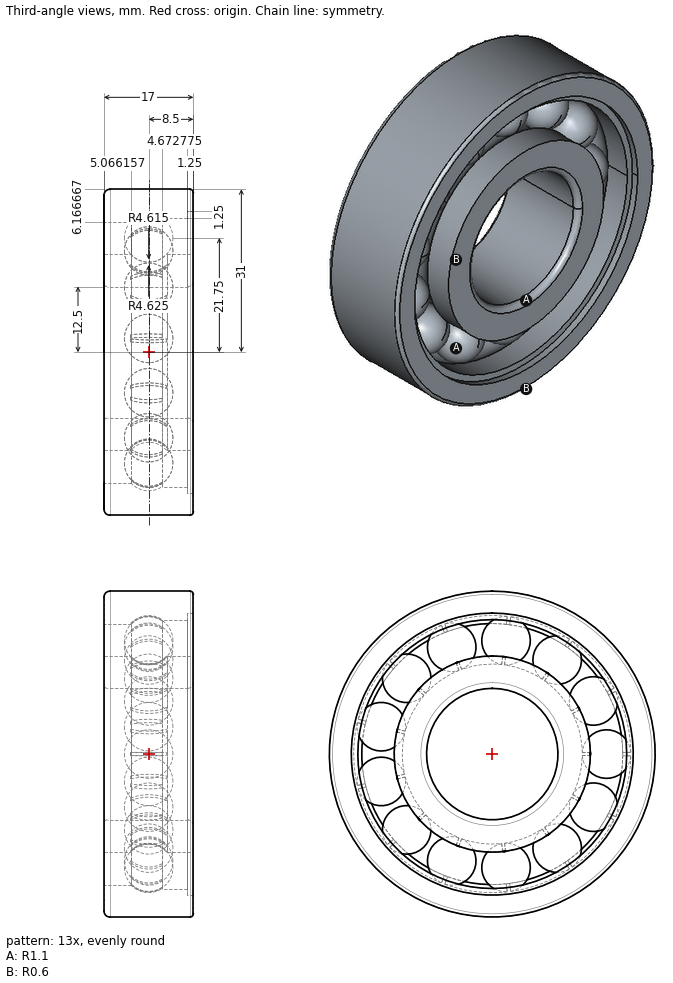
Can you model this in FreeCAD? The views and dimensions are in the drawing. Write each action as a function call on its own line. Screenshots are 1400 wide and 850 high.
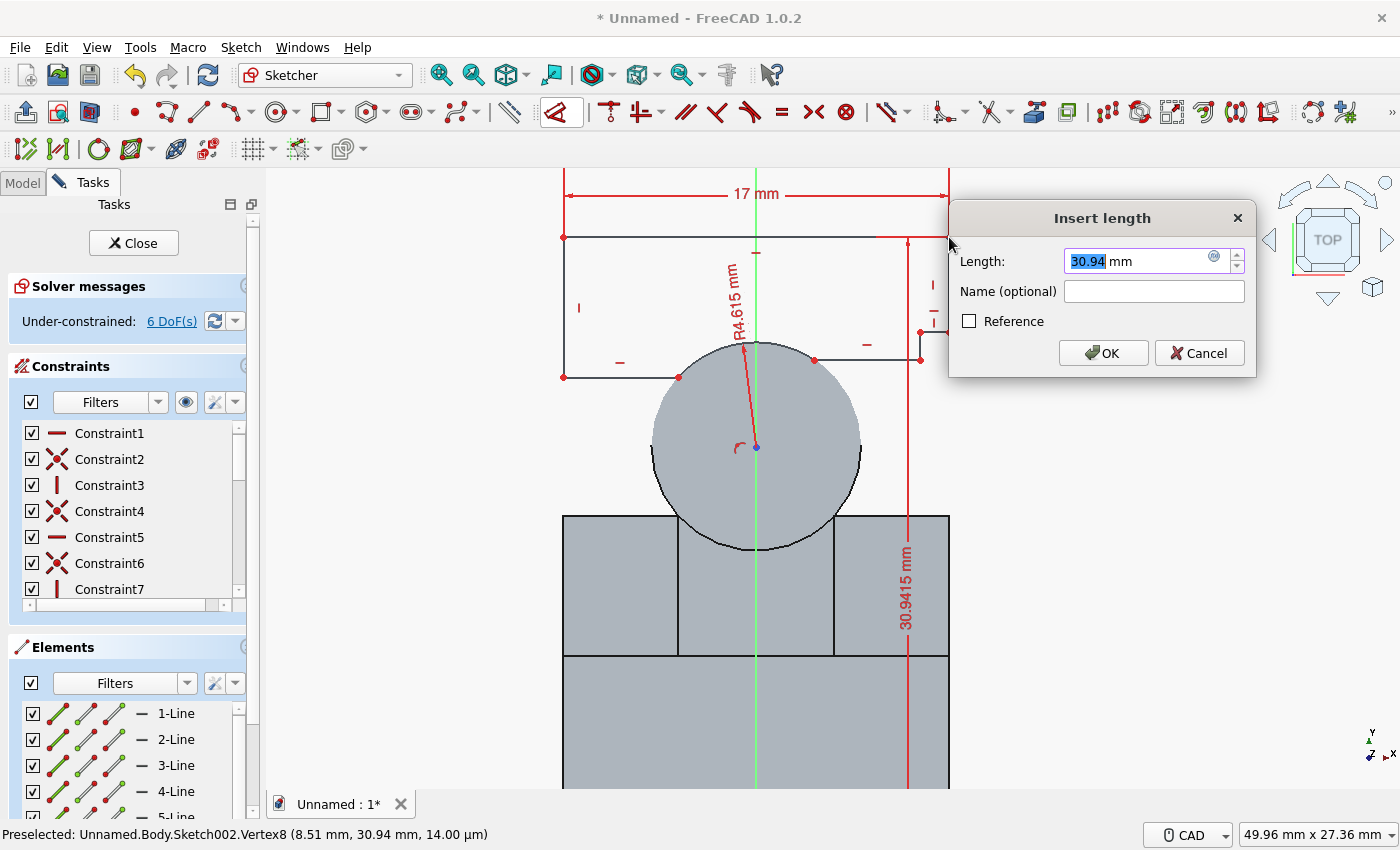
text(31)
key(Return)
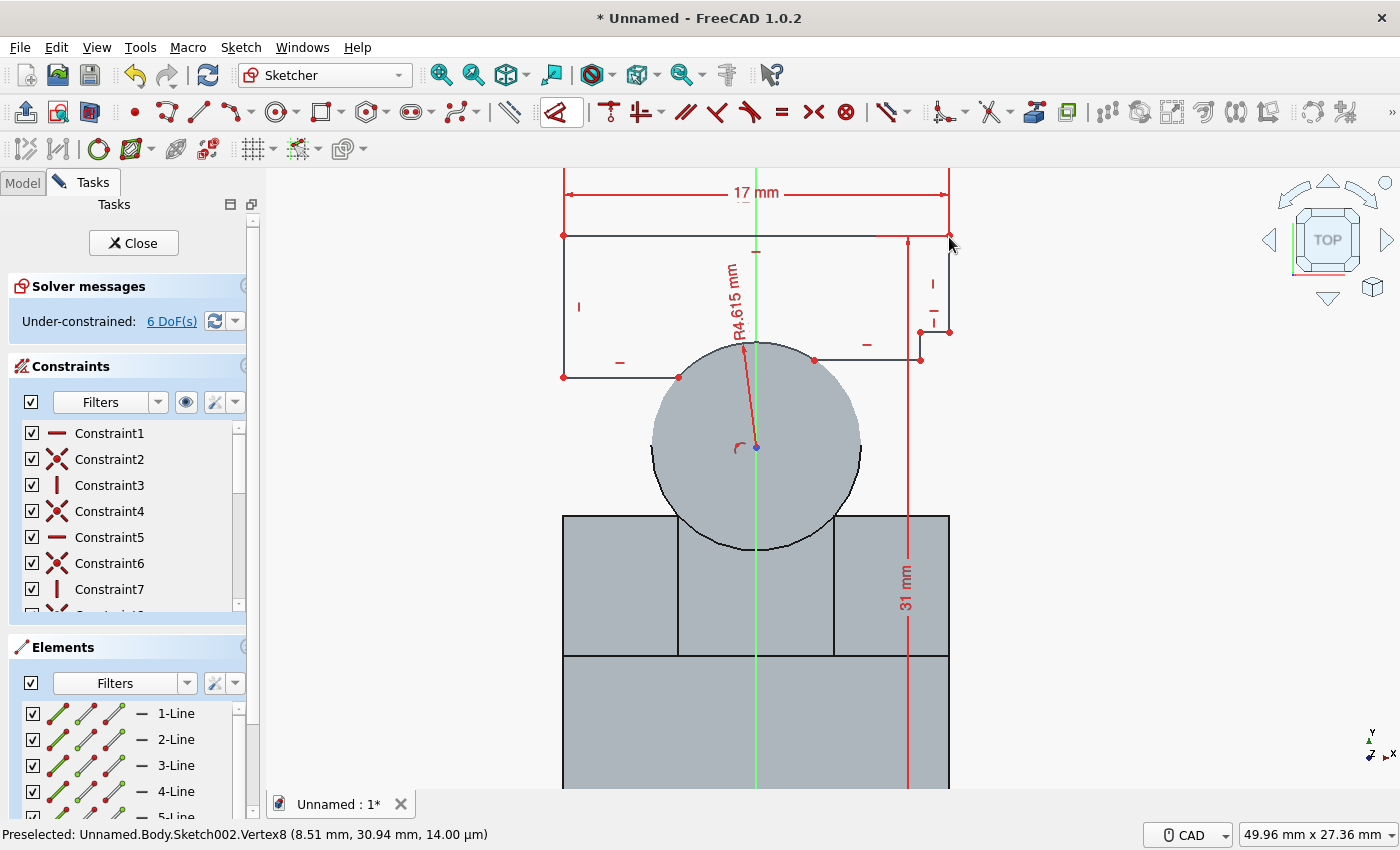
scroll(920, 349, up, 2)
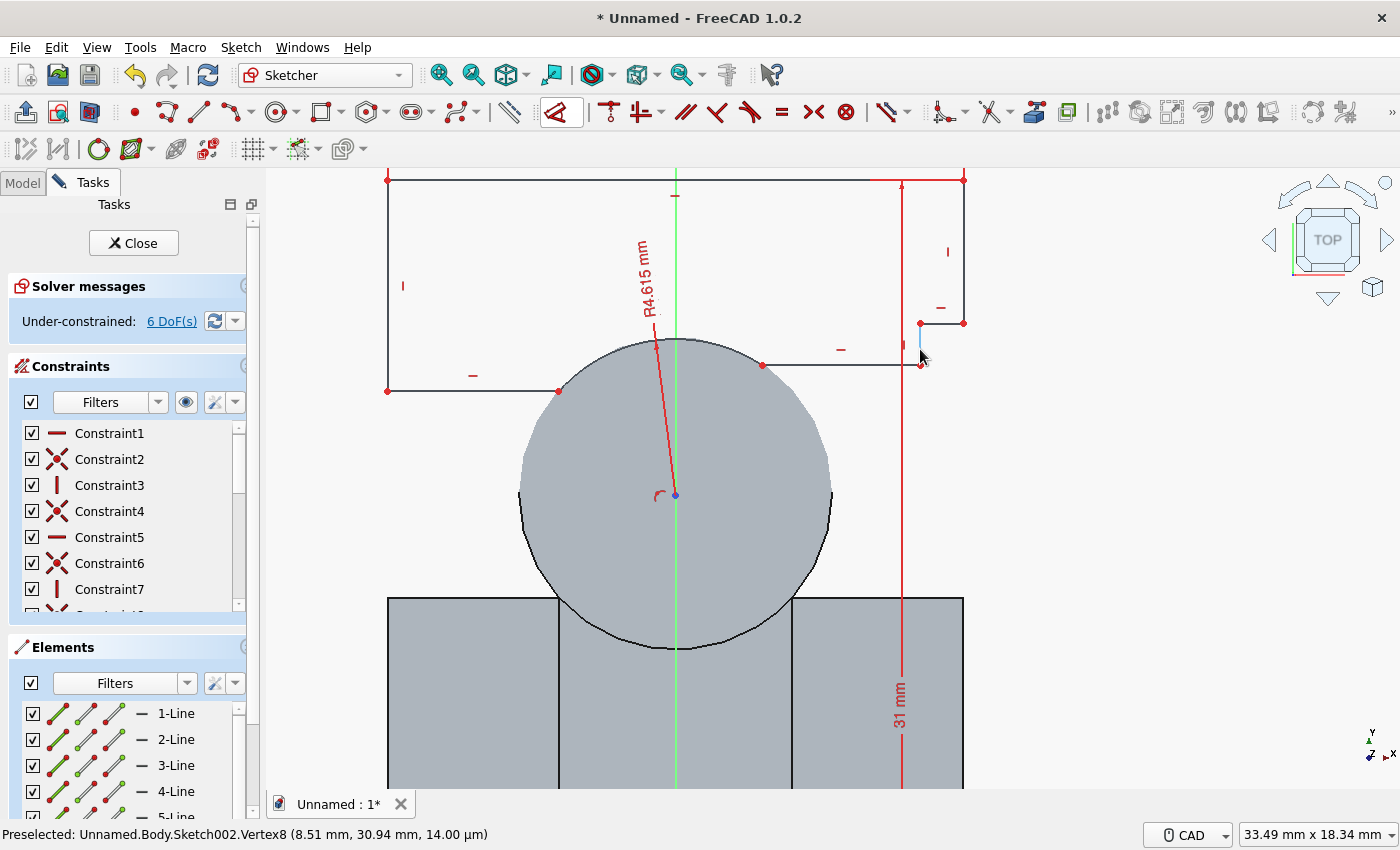
click(920, 349)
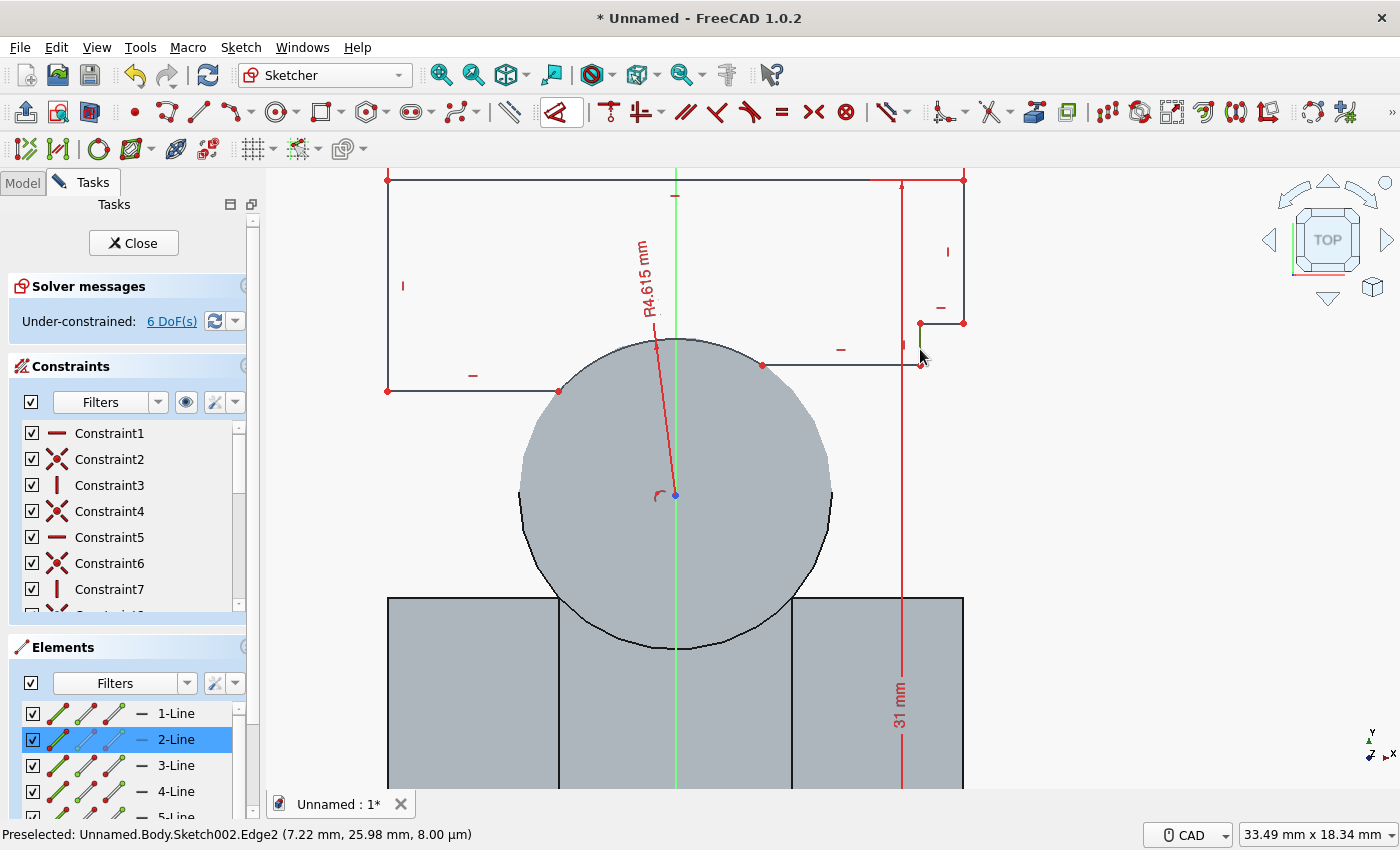
click(578, 112)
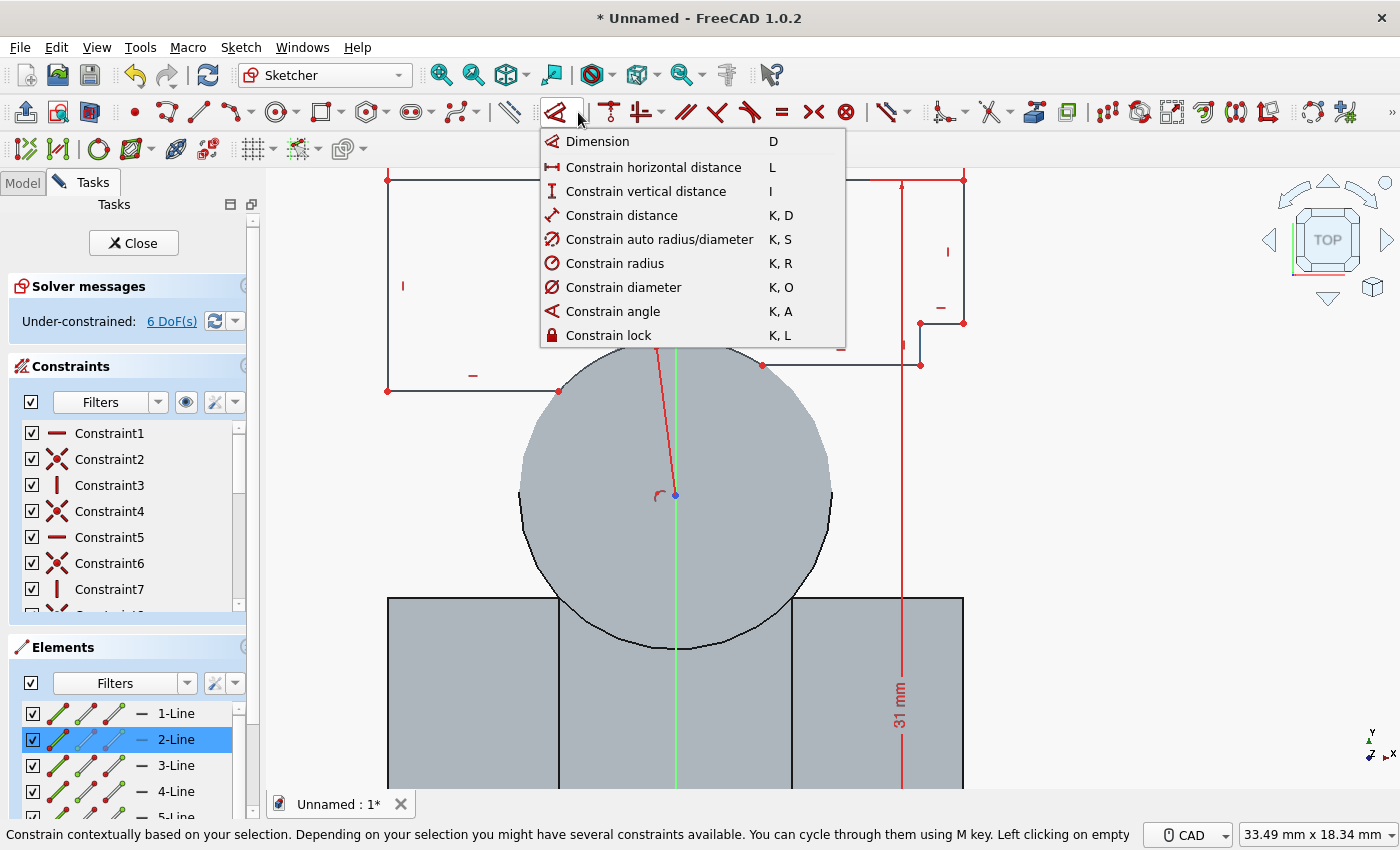
click(693, 191)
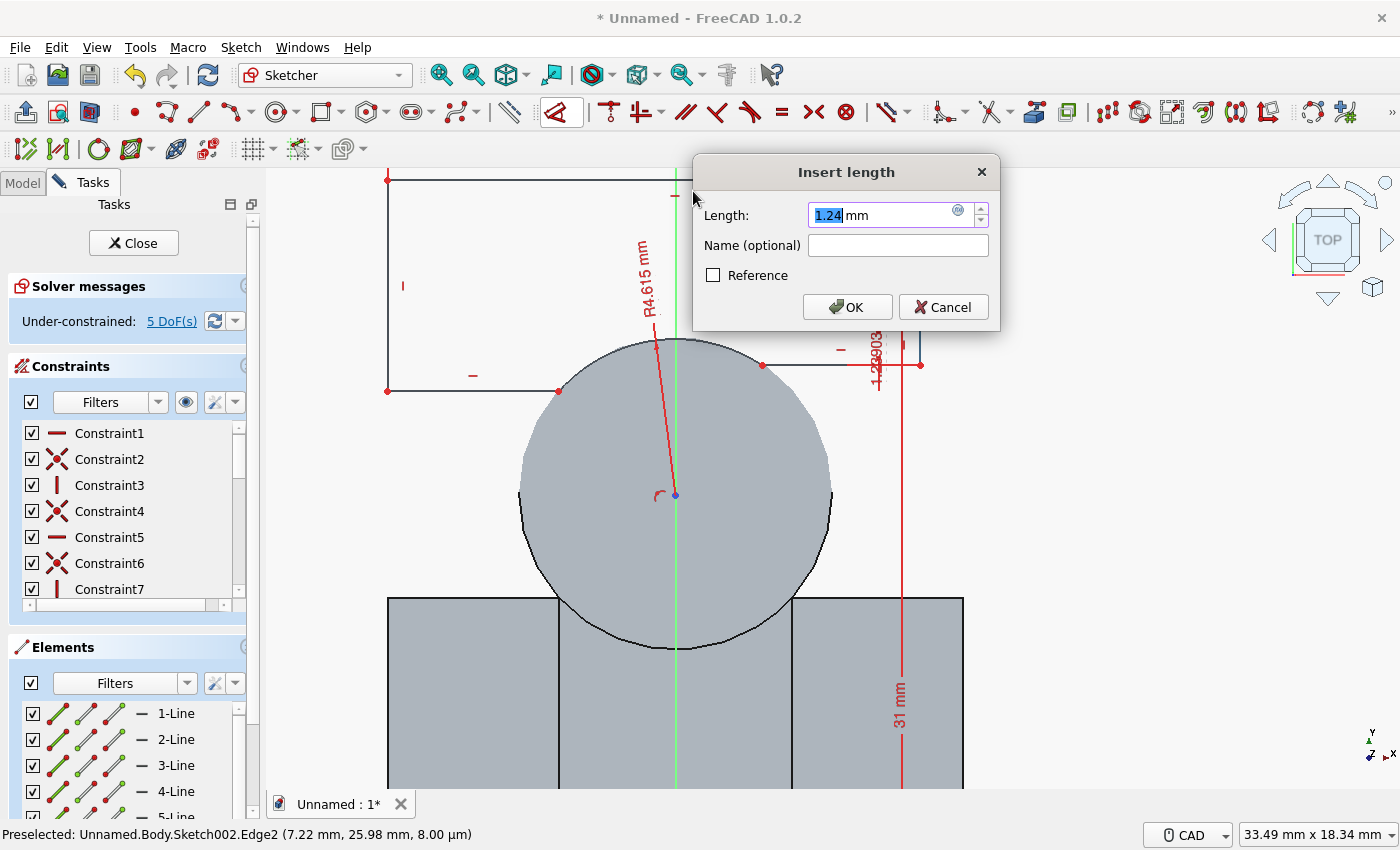
text(1.25)
key(Return)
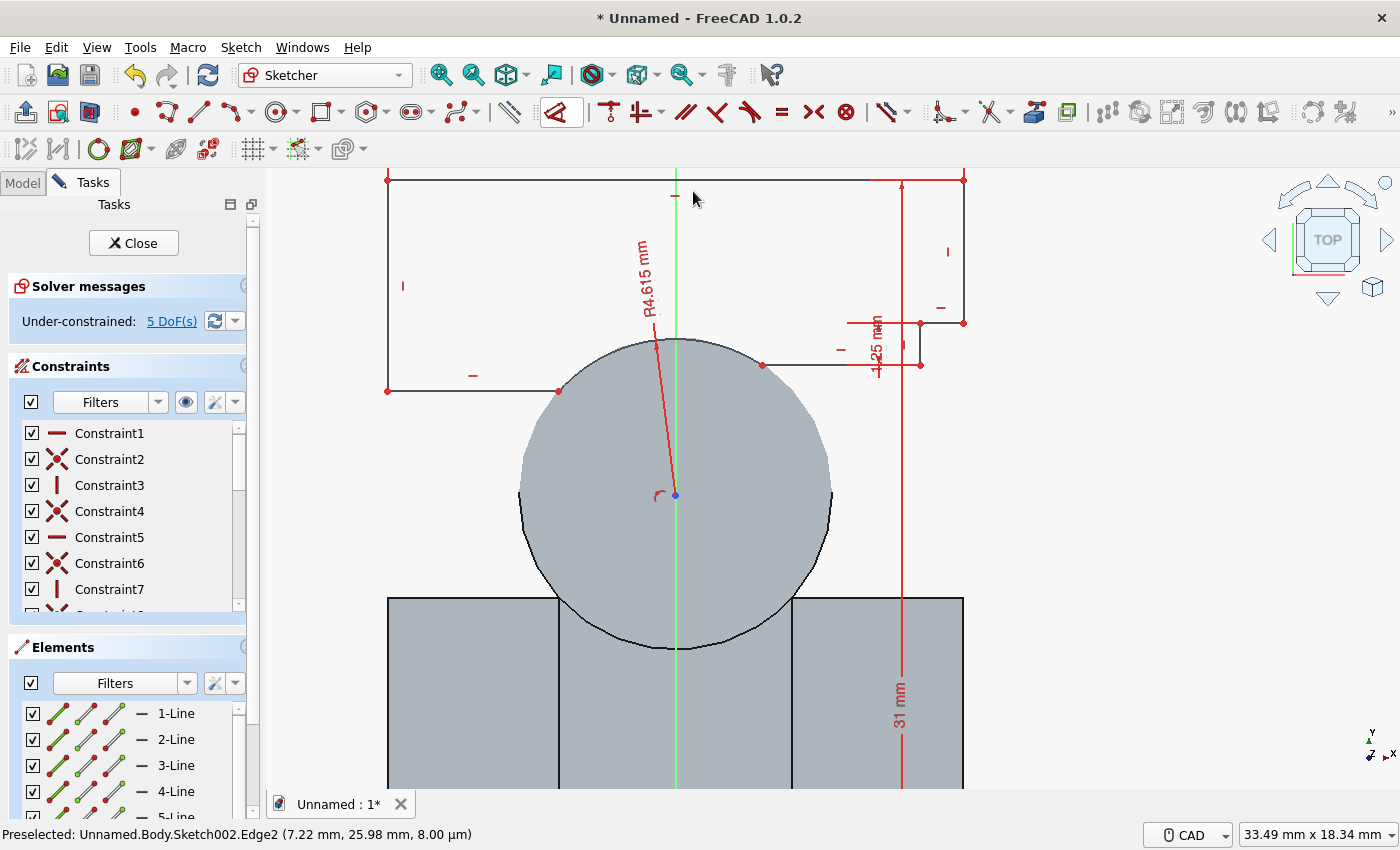
click(933, 323)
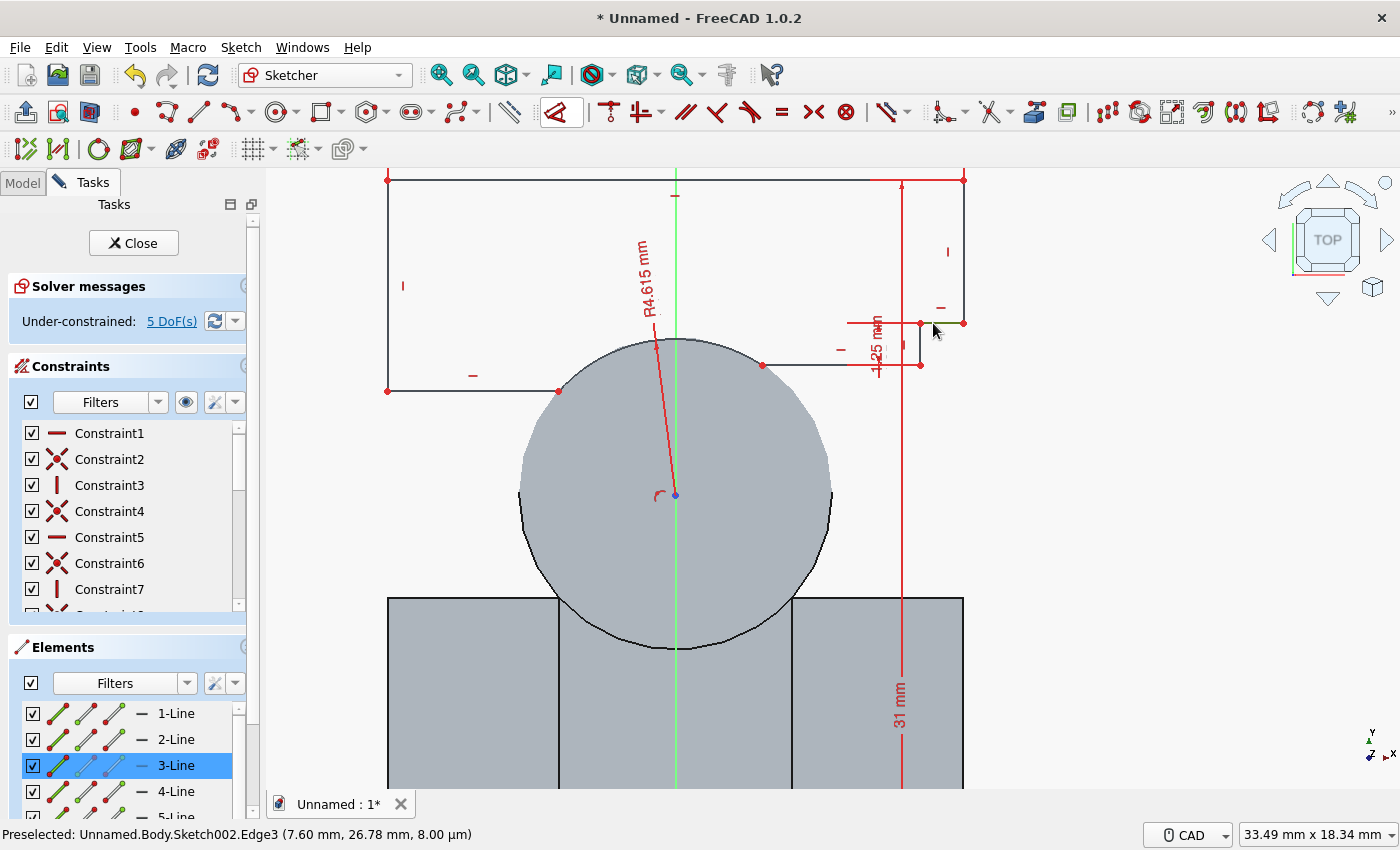
key(l)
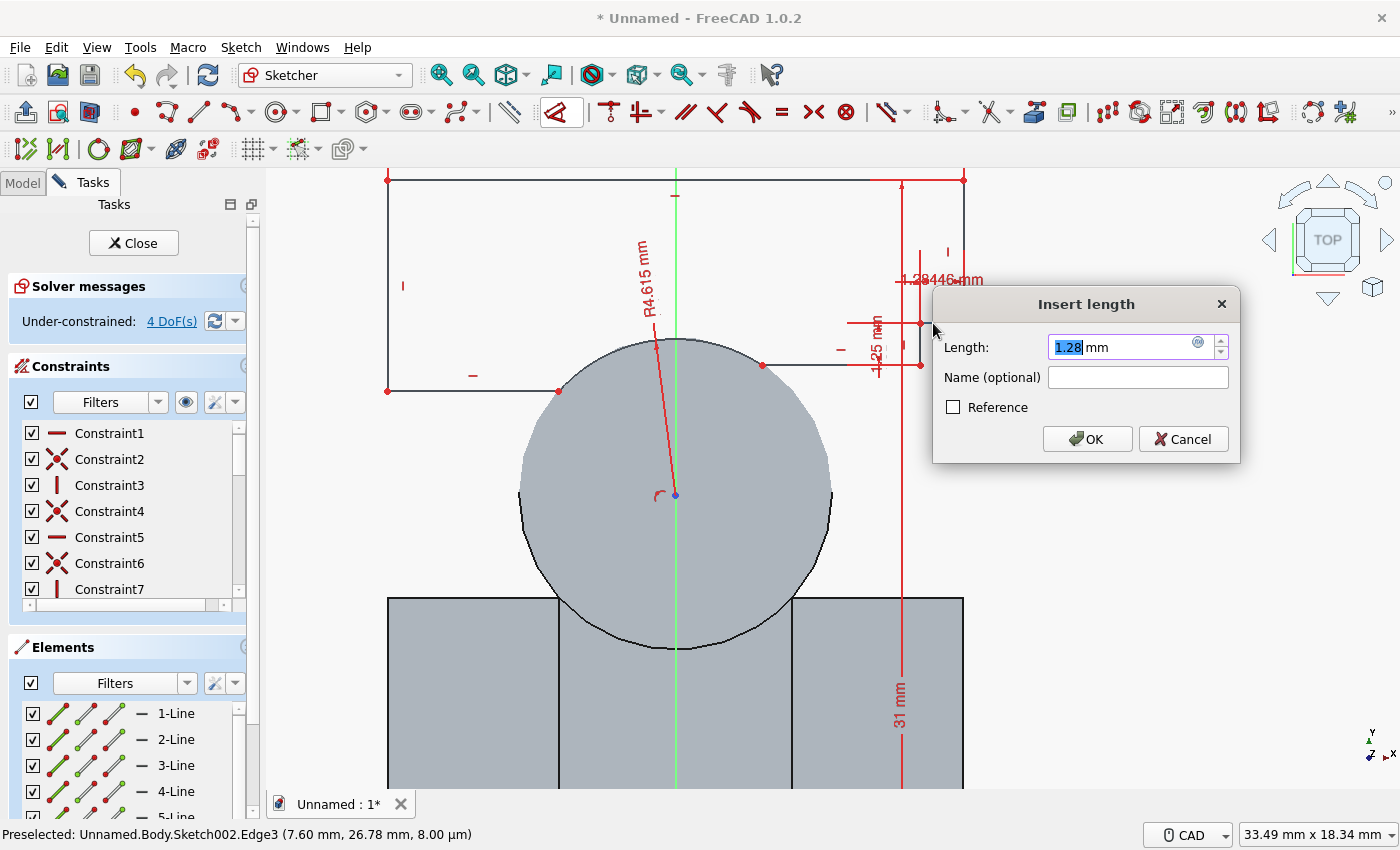
text(1.25)
key(Return)